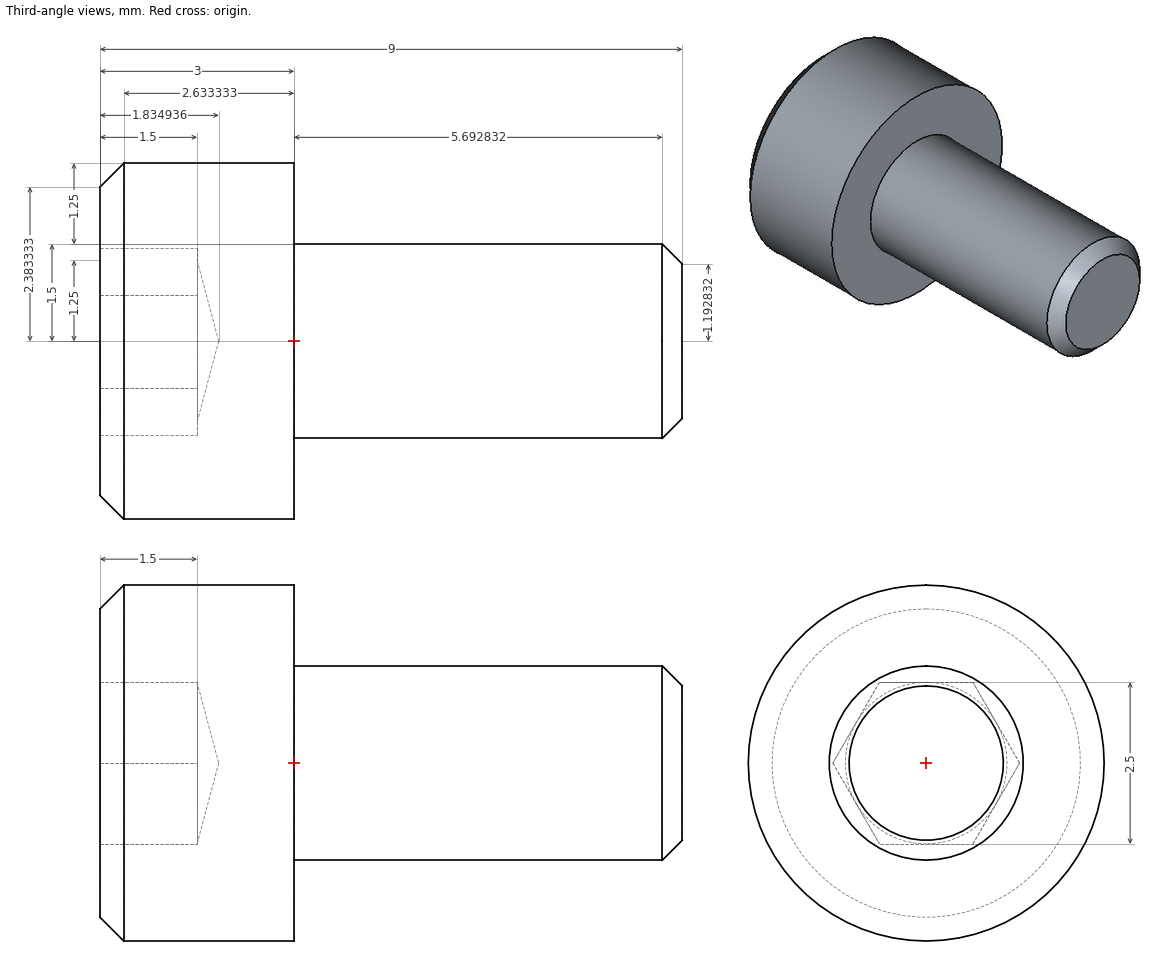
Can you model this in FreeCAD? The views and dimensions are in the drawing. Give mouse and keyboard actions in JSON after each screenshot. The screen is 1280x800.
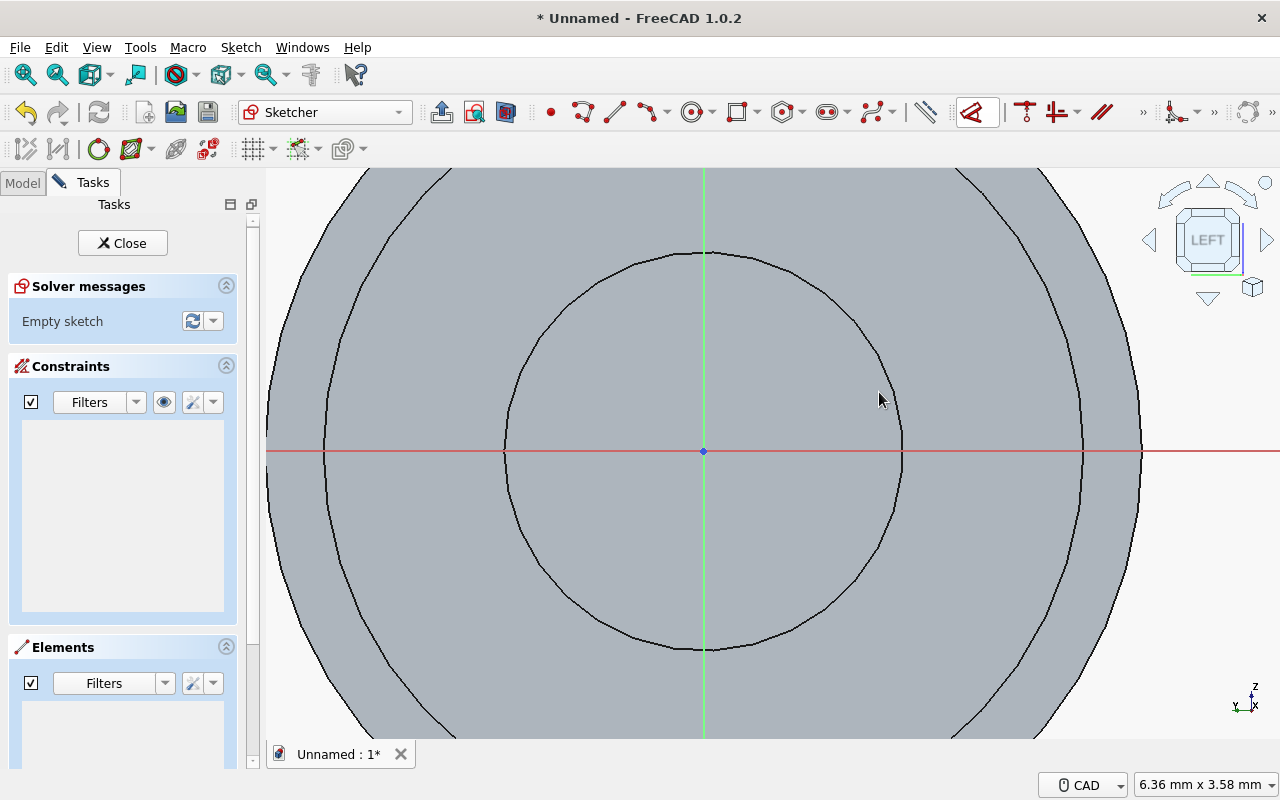
{"action": "key", "text": "g p 6"}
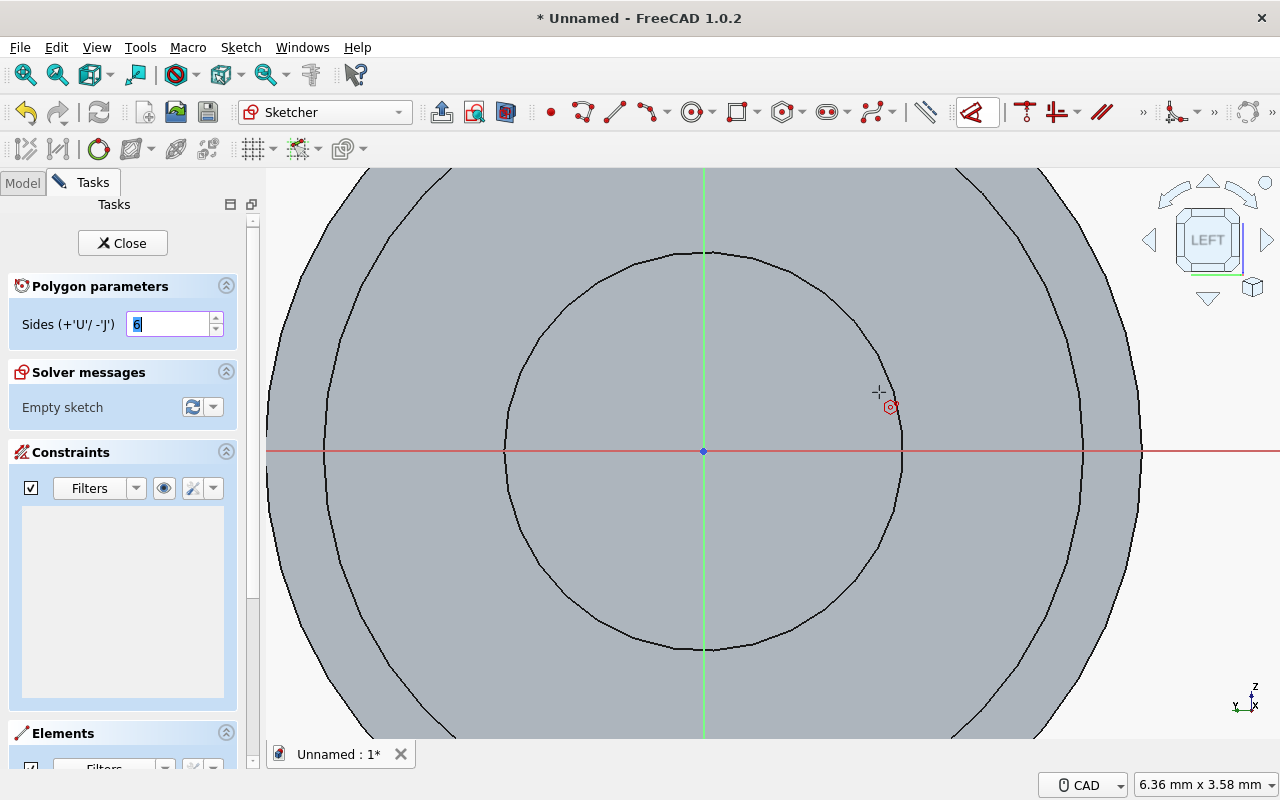
{"action": "left_click", "coordinate": [704, 451]}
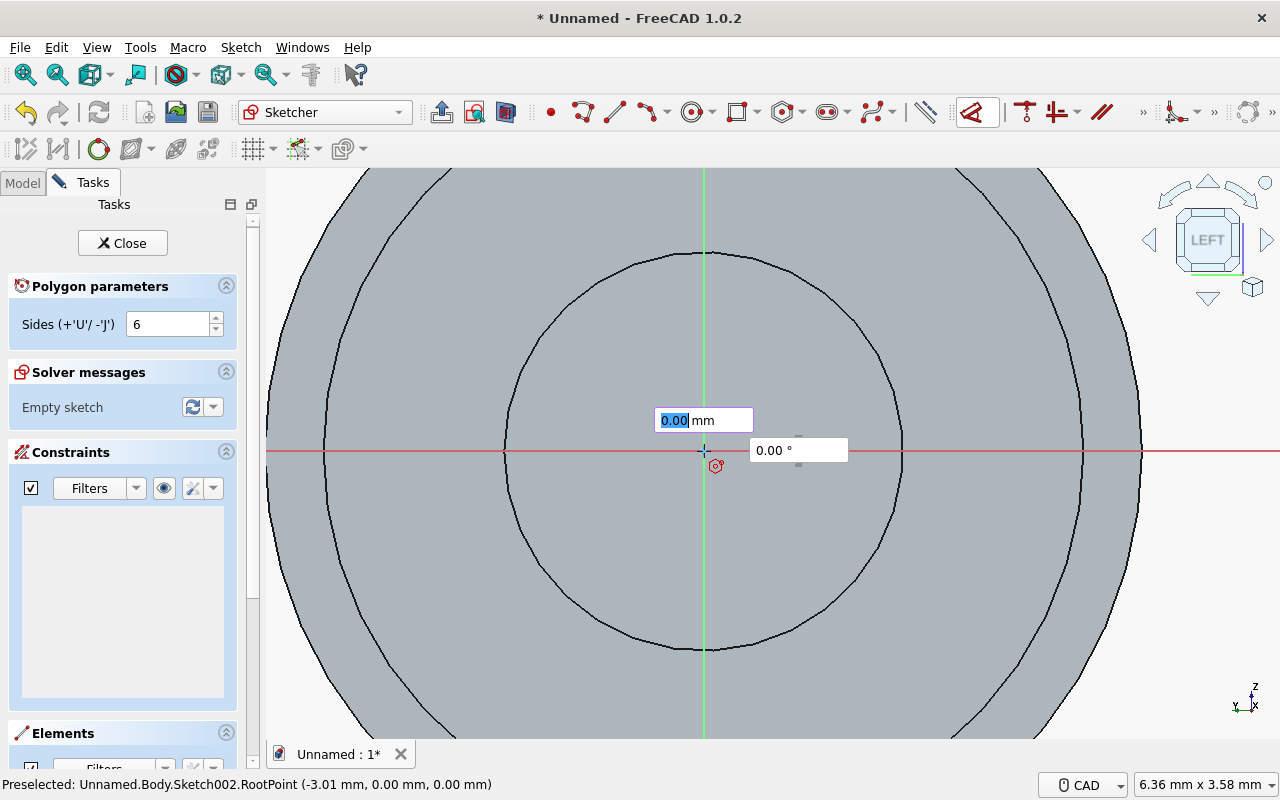
{"action": "left_click", "coordinate": [934, 451]}
{"action": "right_click", "coordinate": [934, 451]}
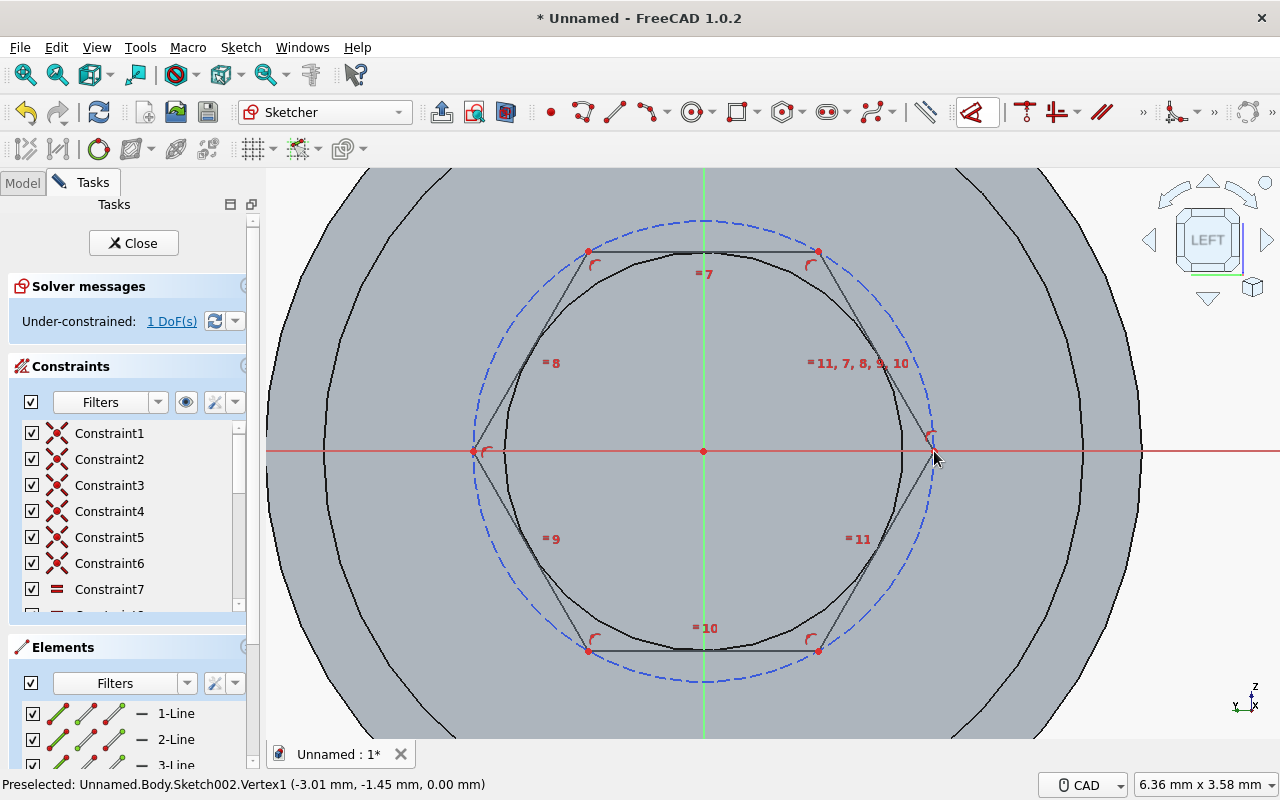
{"action": "left_click", "coordinate": [588, 651]}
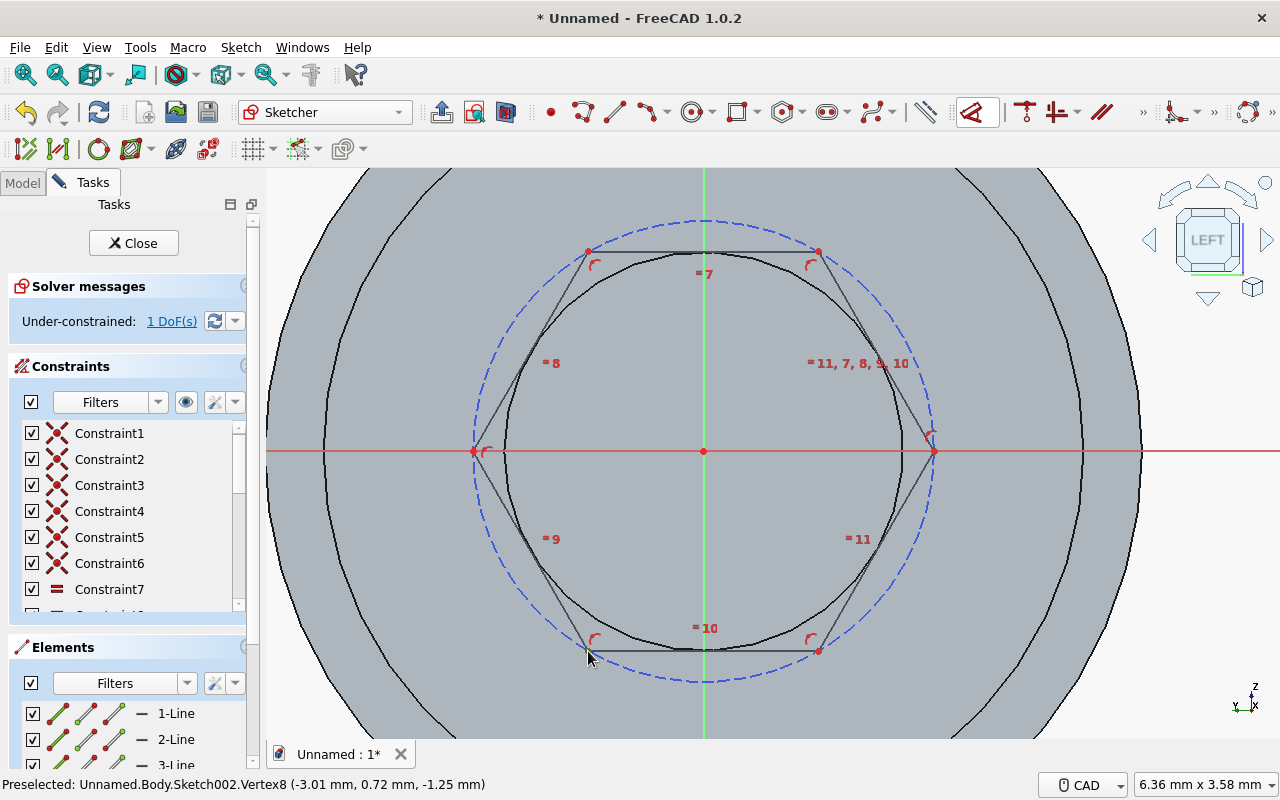
{"action": "left_click", "coordinate": [819, 252]}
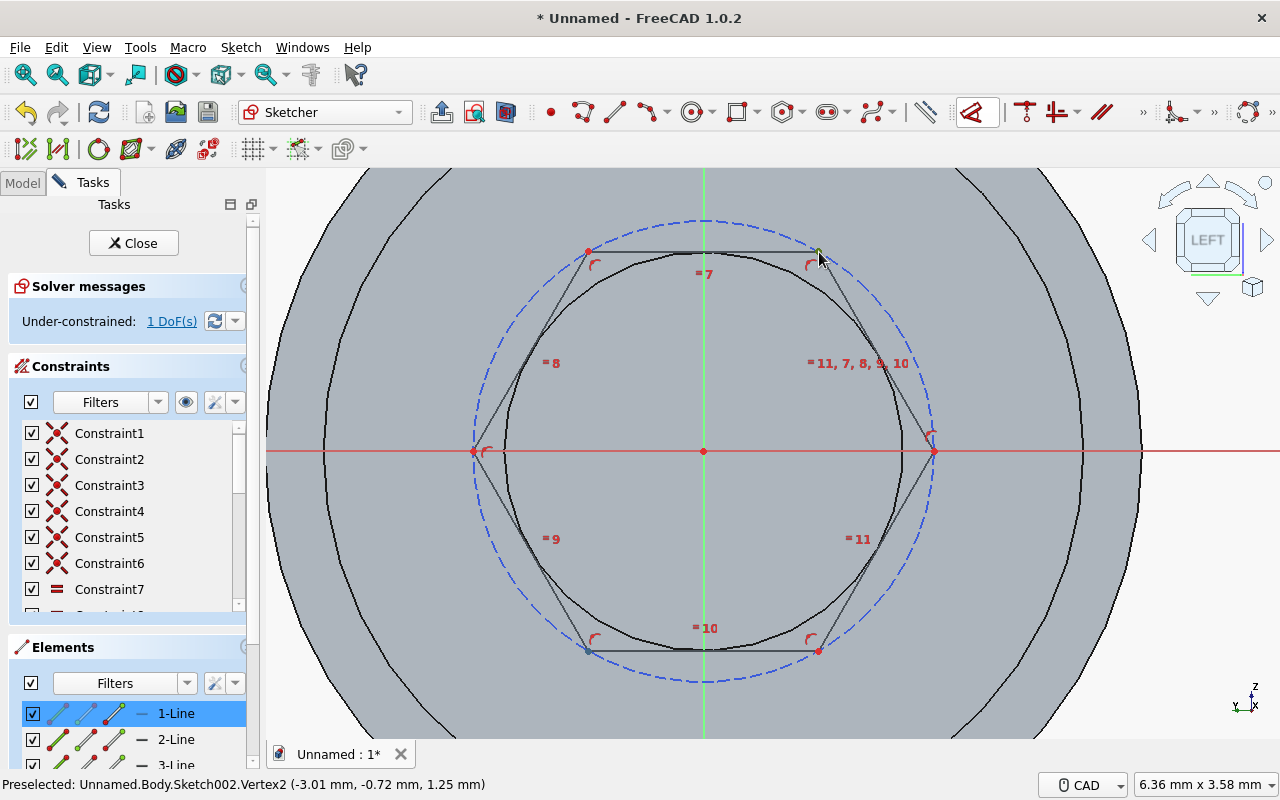
{"action": "key", "text": "i"}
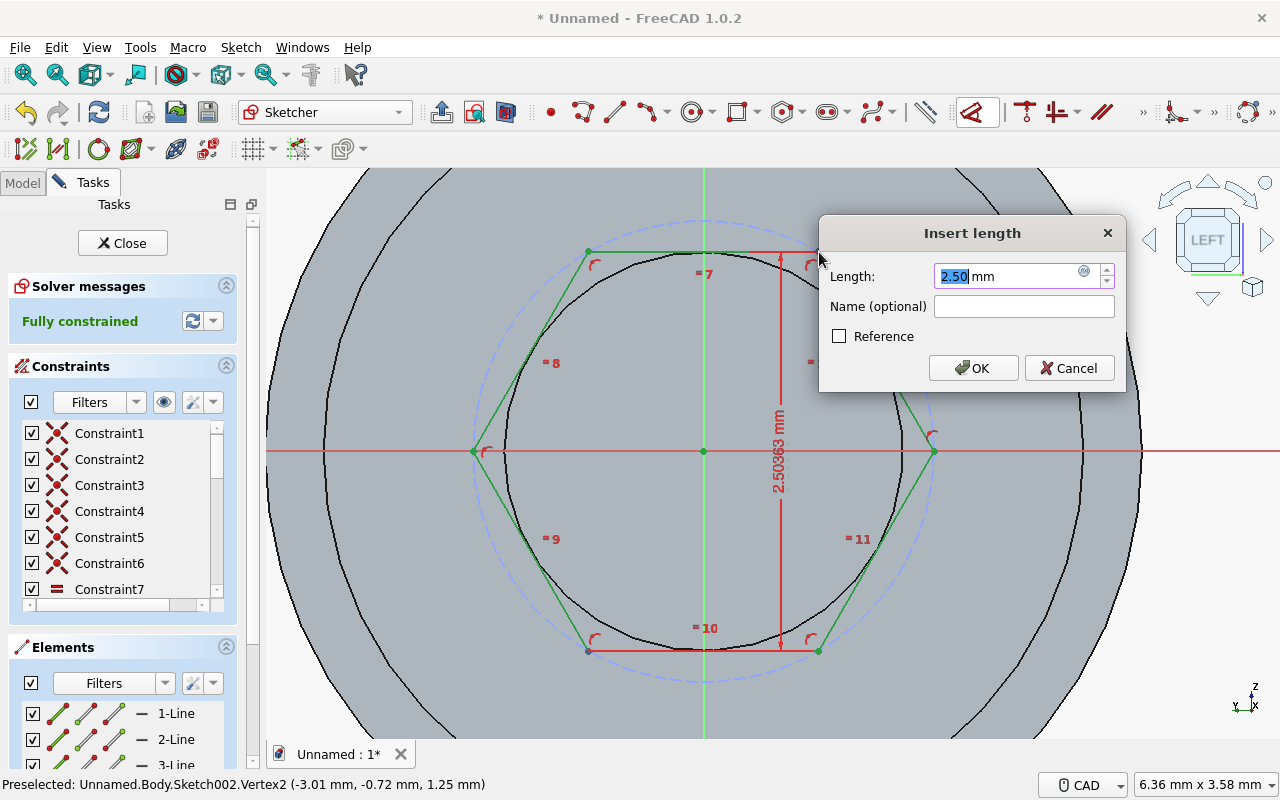
{"action": "type", "text": "2.5"}
{"action": "key", "text": "Return"}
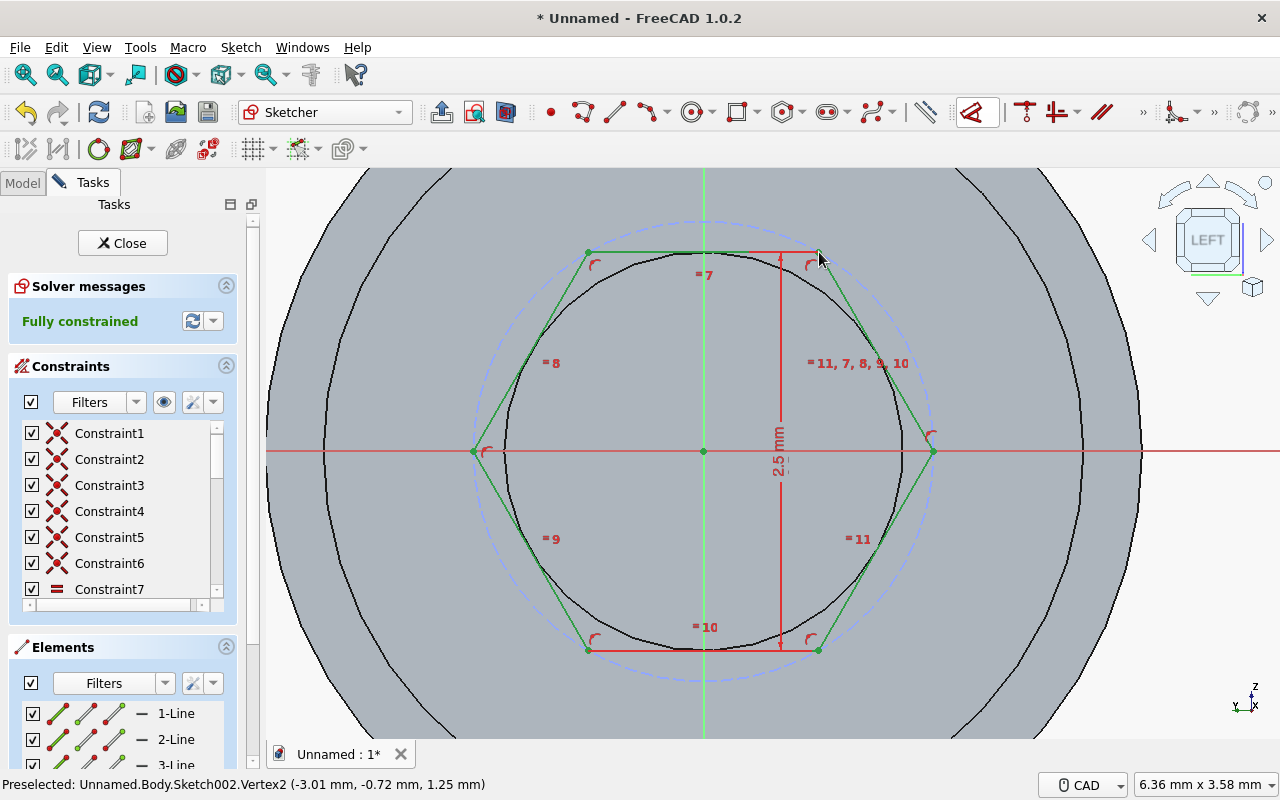
{"action": "left_click", "coordinate": [123, 243]}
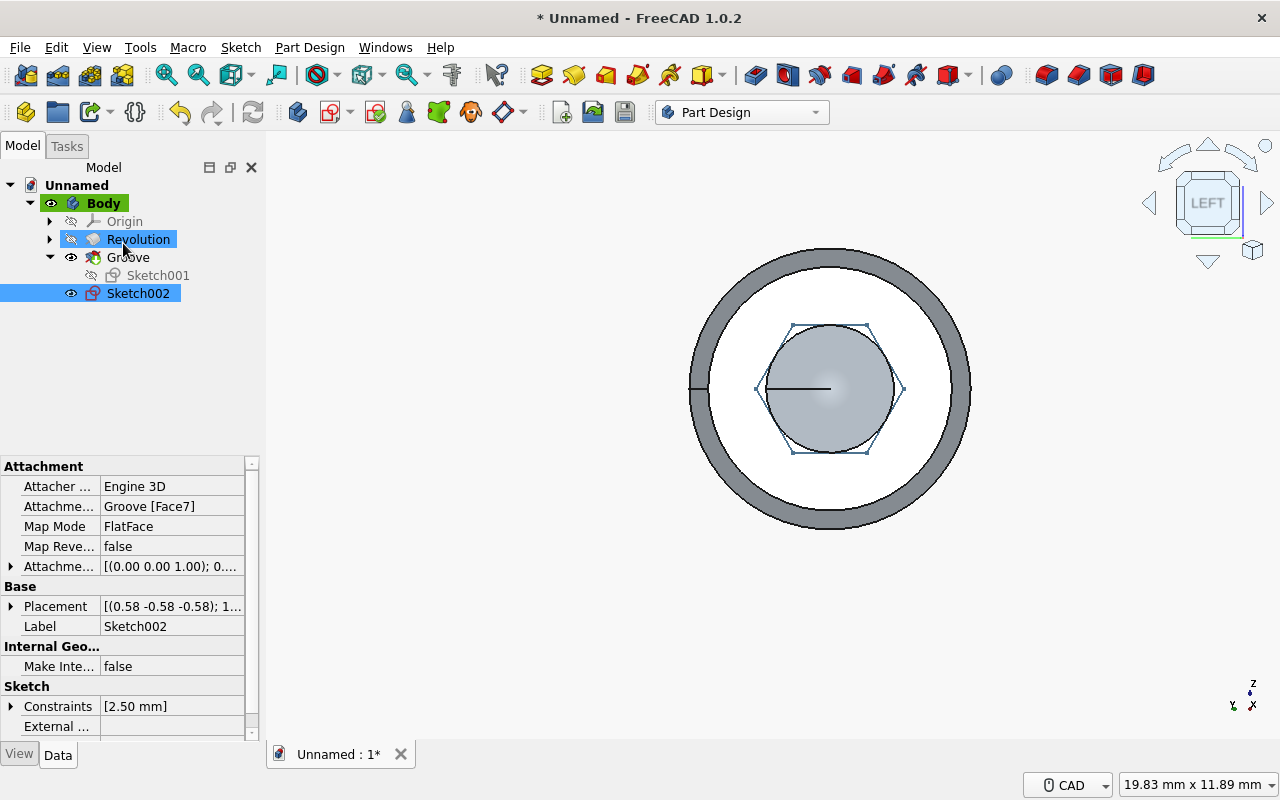
{"action": "left_click", "coordinate": [756, 76]}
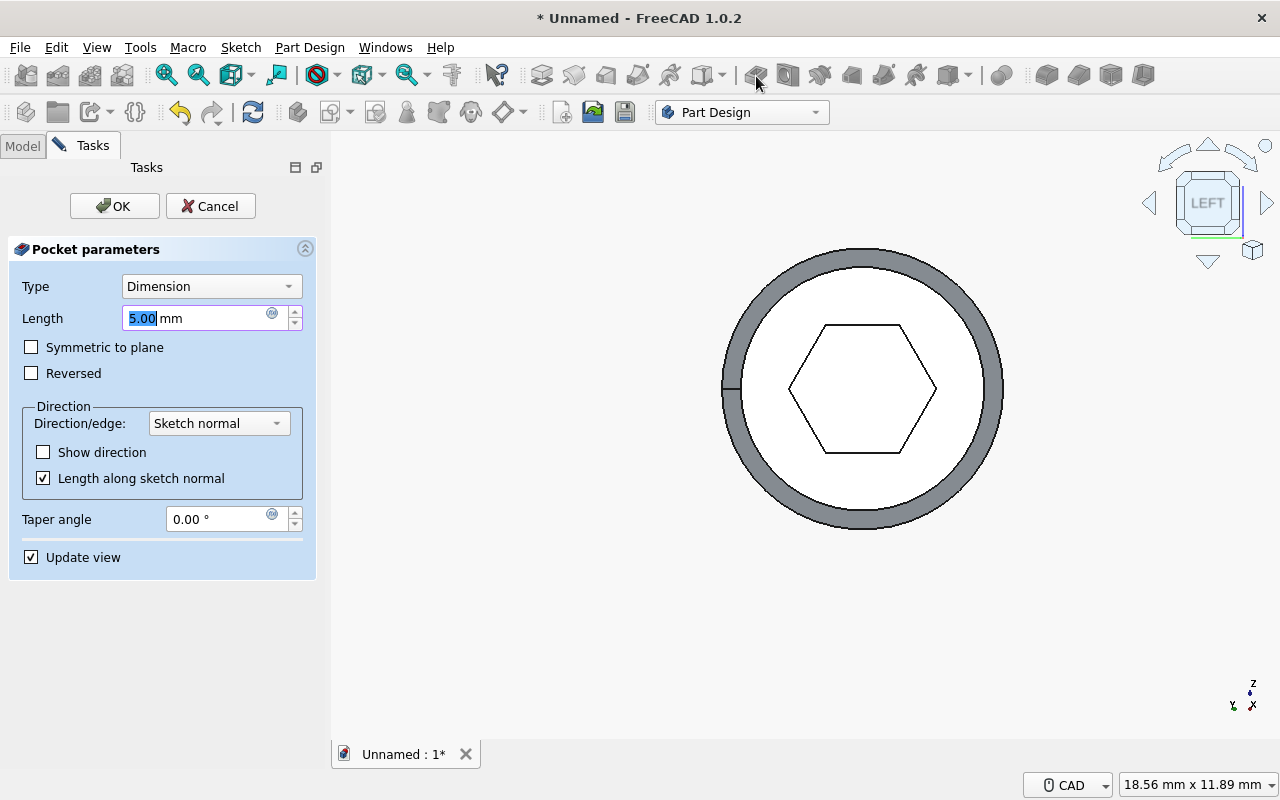
{"action": "type", "text": "1.5"}
{"action": "key", "text": "Tab"}